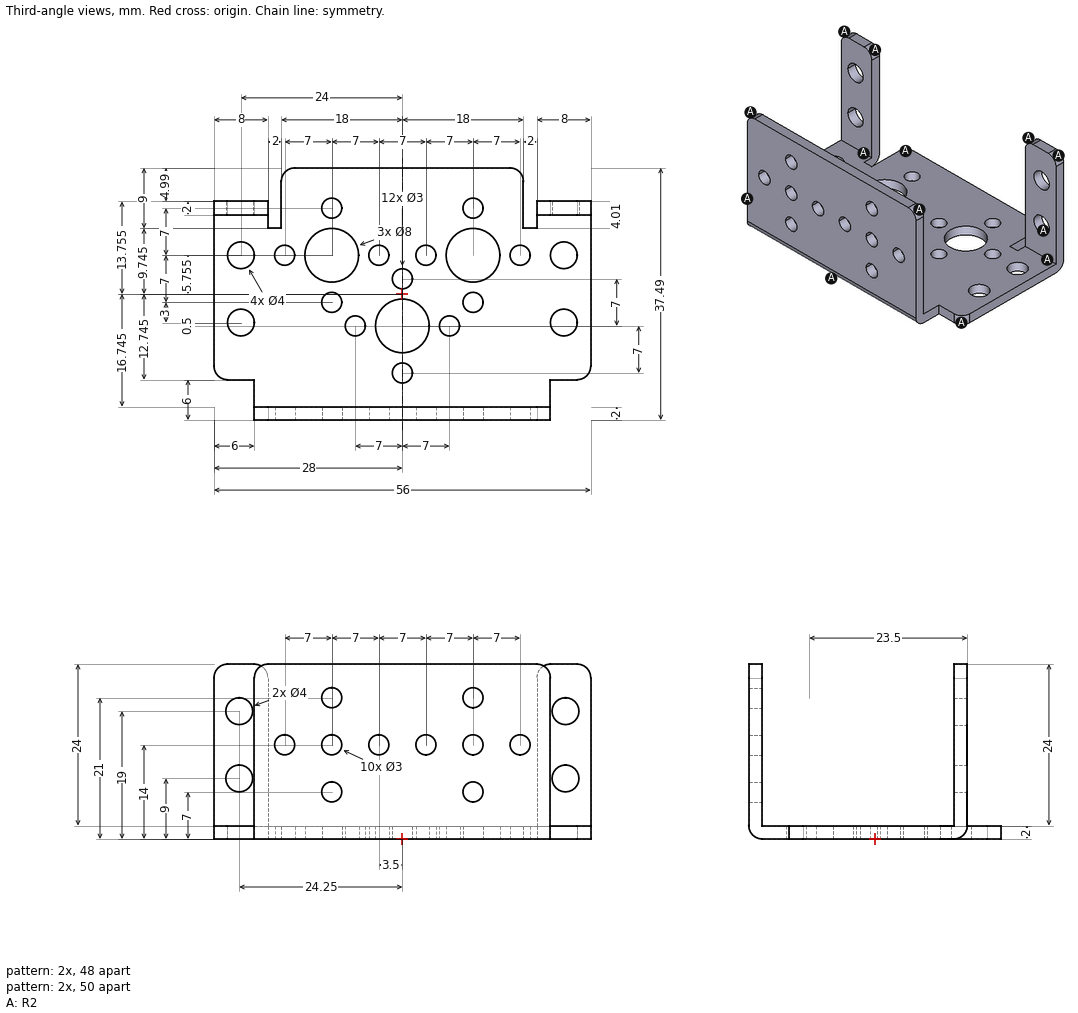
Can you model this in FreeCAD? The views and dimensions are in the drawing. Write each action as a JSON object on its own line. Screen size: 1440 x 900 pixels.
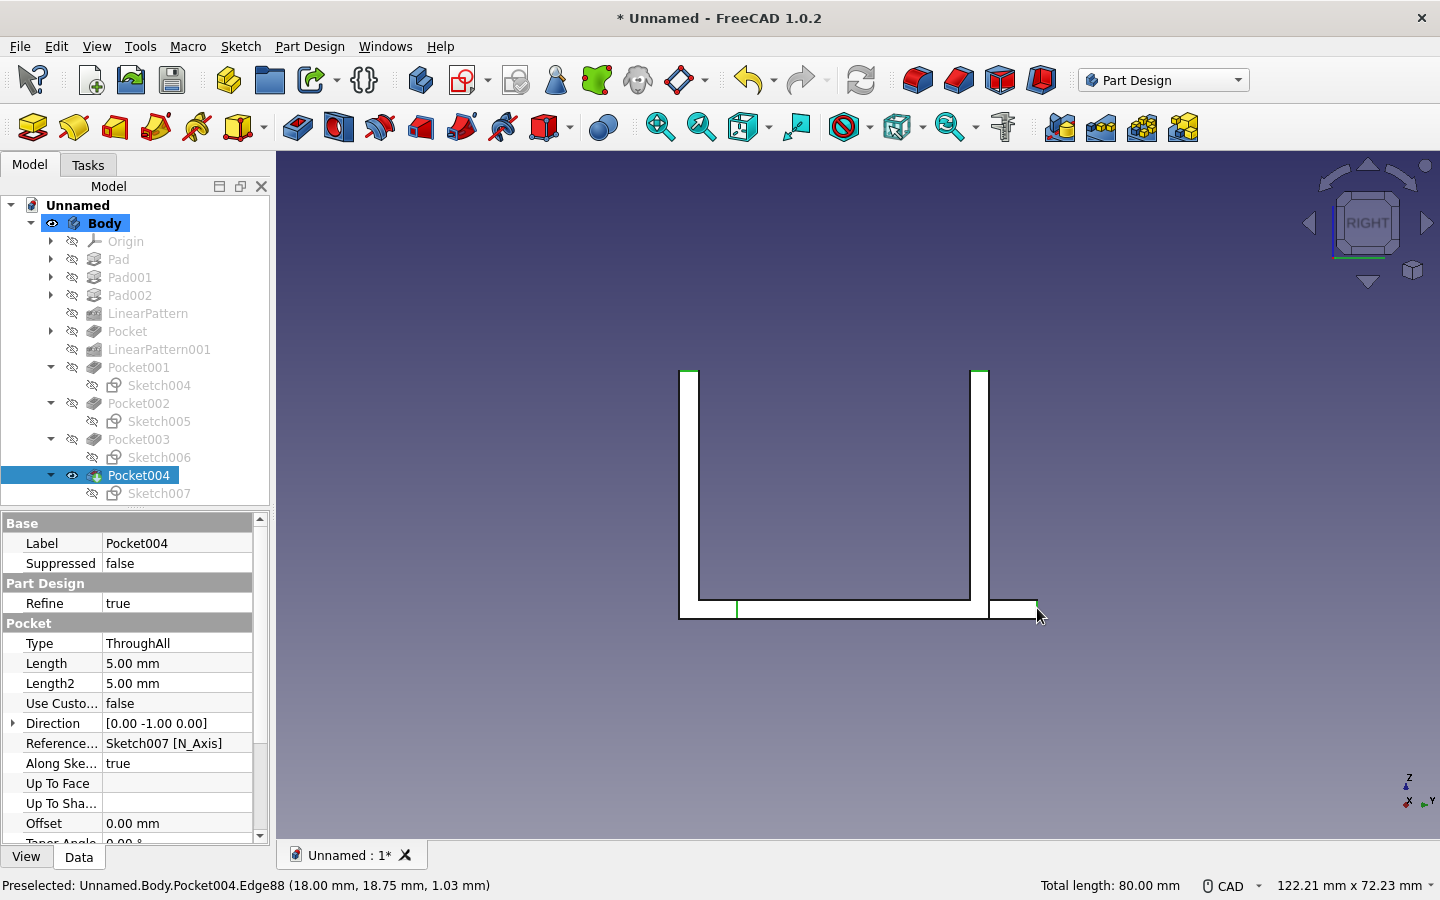
{"action": "left_click", "coordinate": [918, 80]}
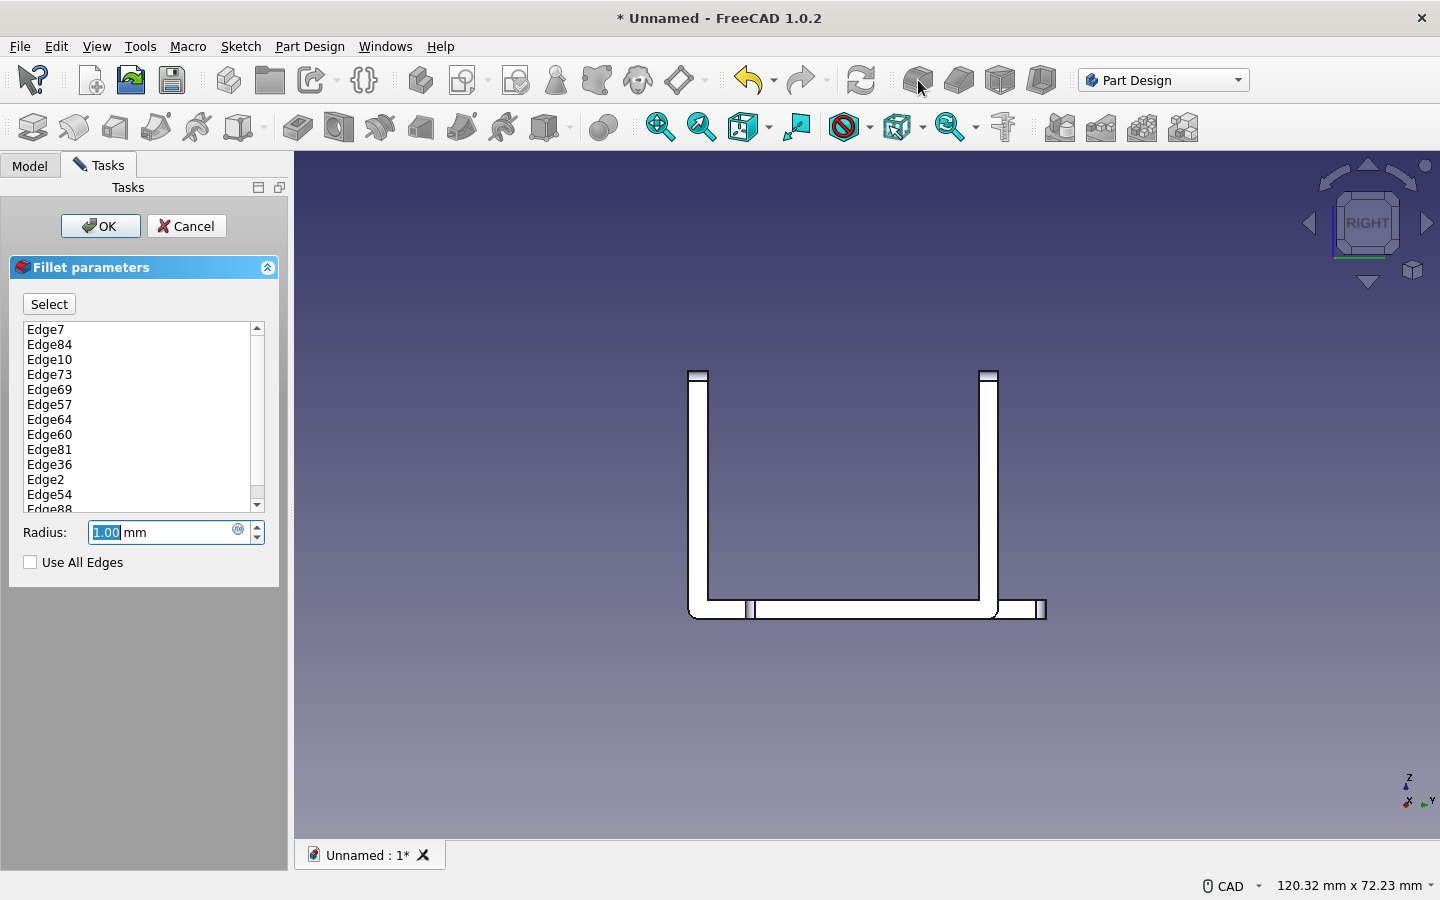
{"action": "type", "text": "2"}
{"action": "key", "text": "Tab"}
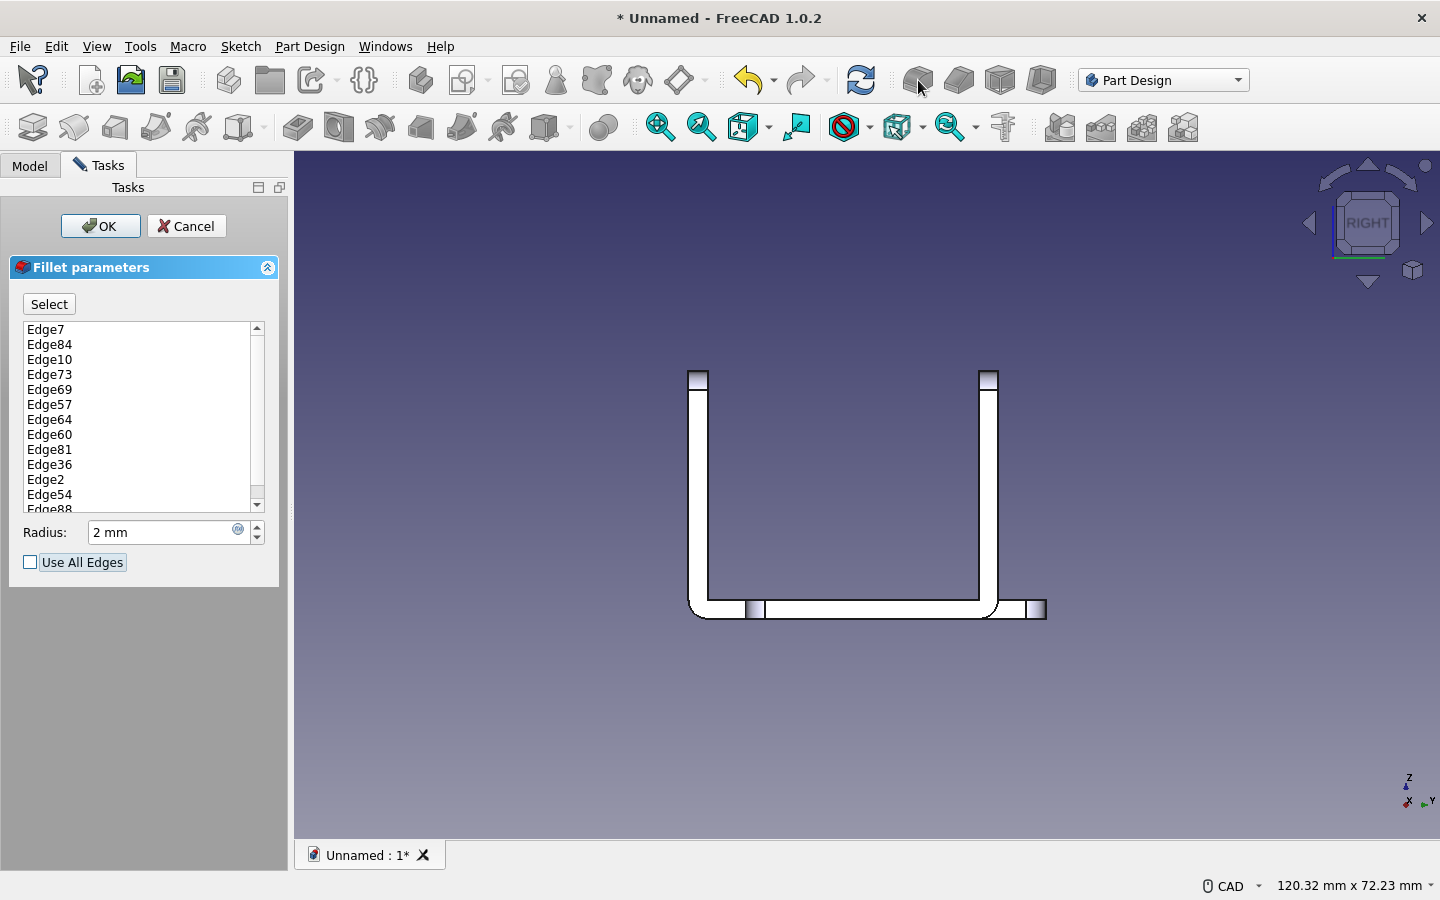
{"action": "left_click", "coordinate": [101, 226]}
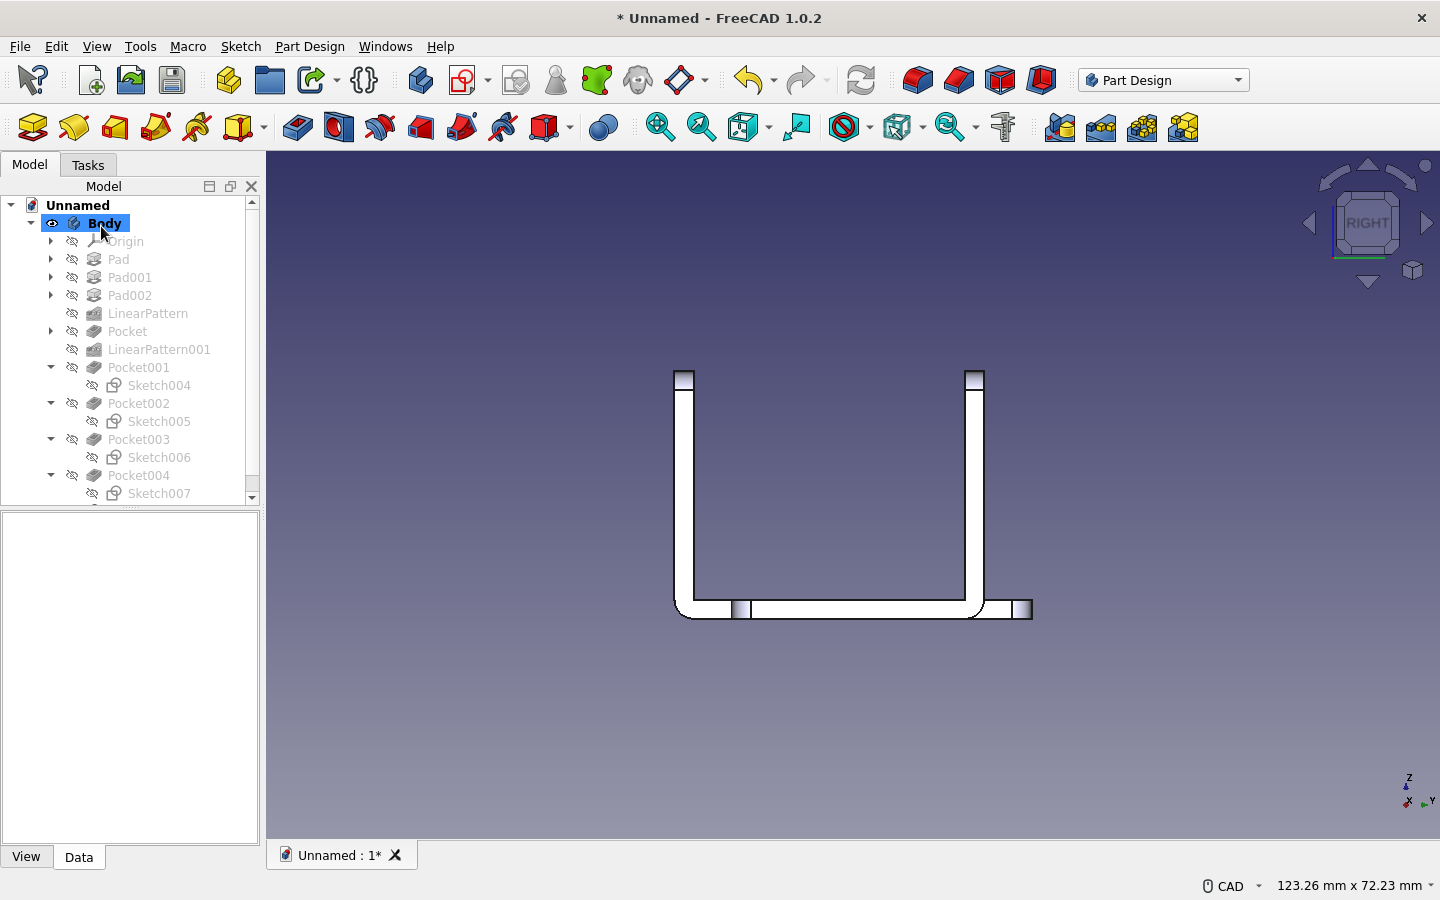
{"action": "key", "text": "v f"}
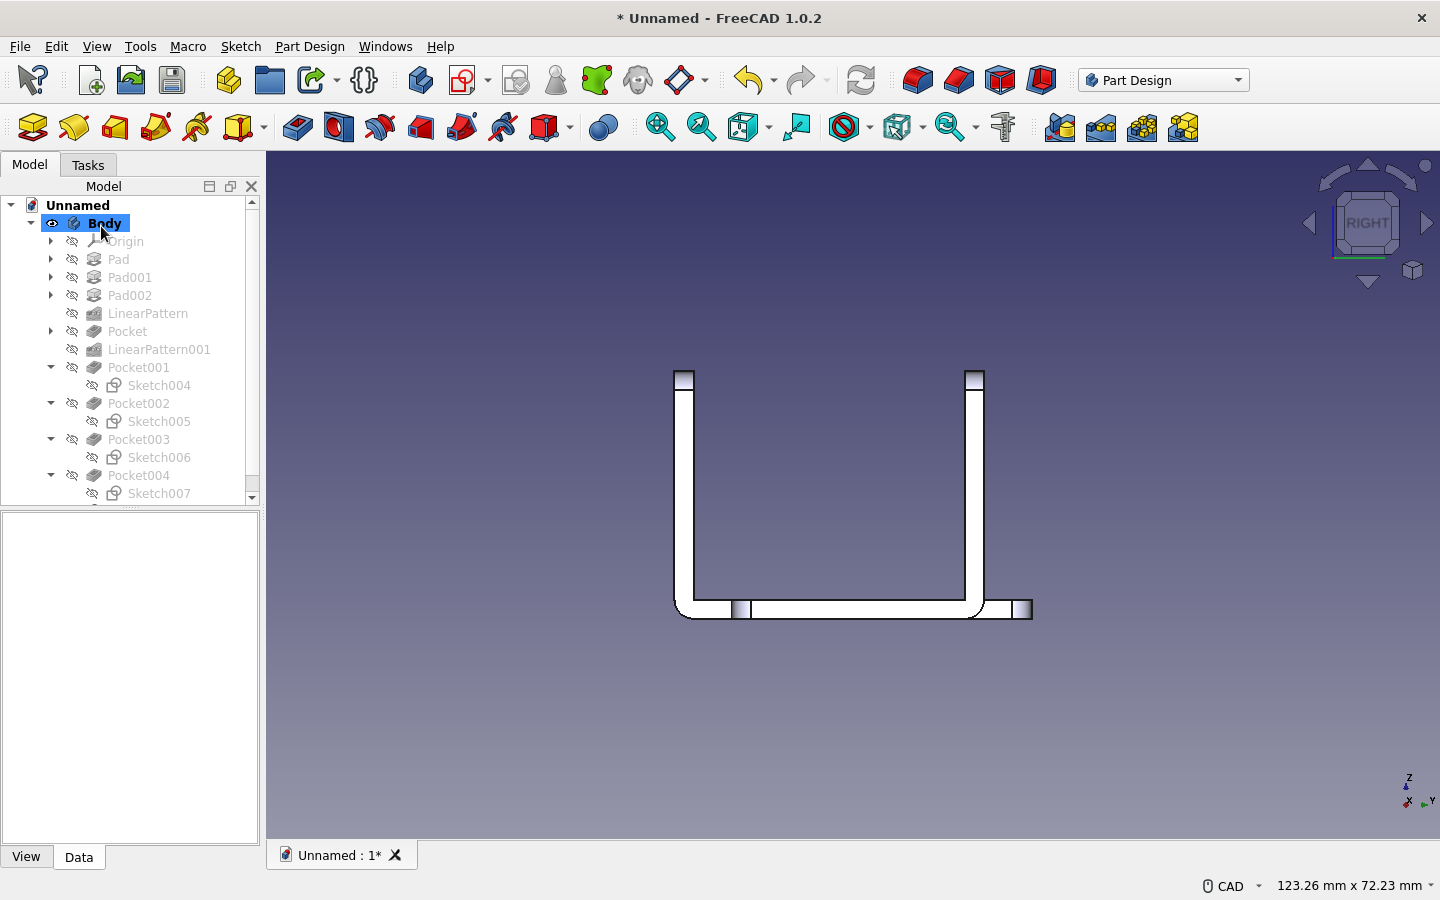
{"action": "key", "text": "4"}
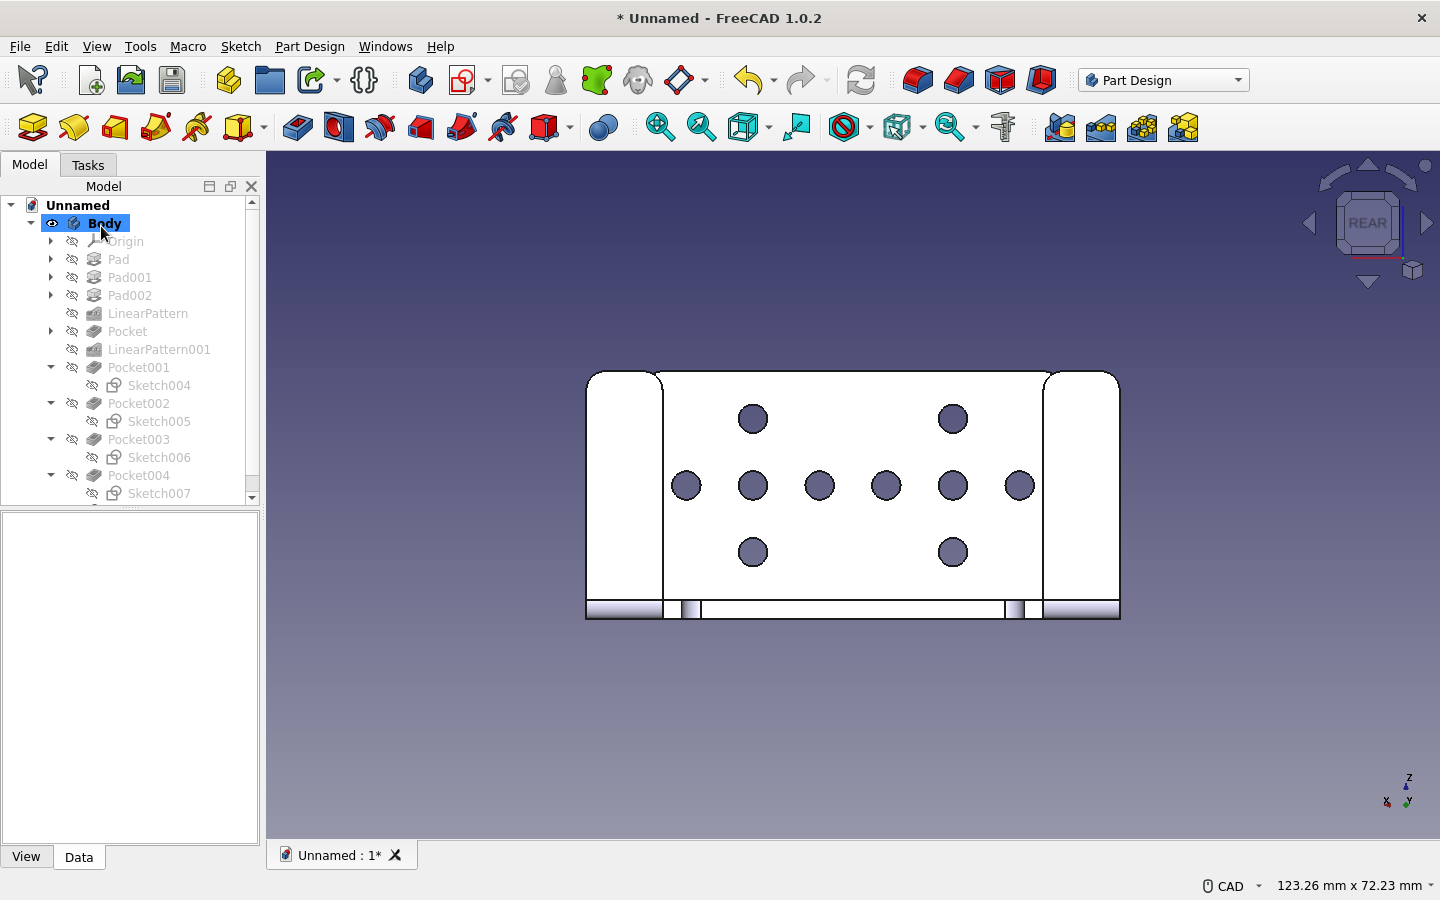
{"action": "left_click", "coordinate": [624, 419]}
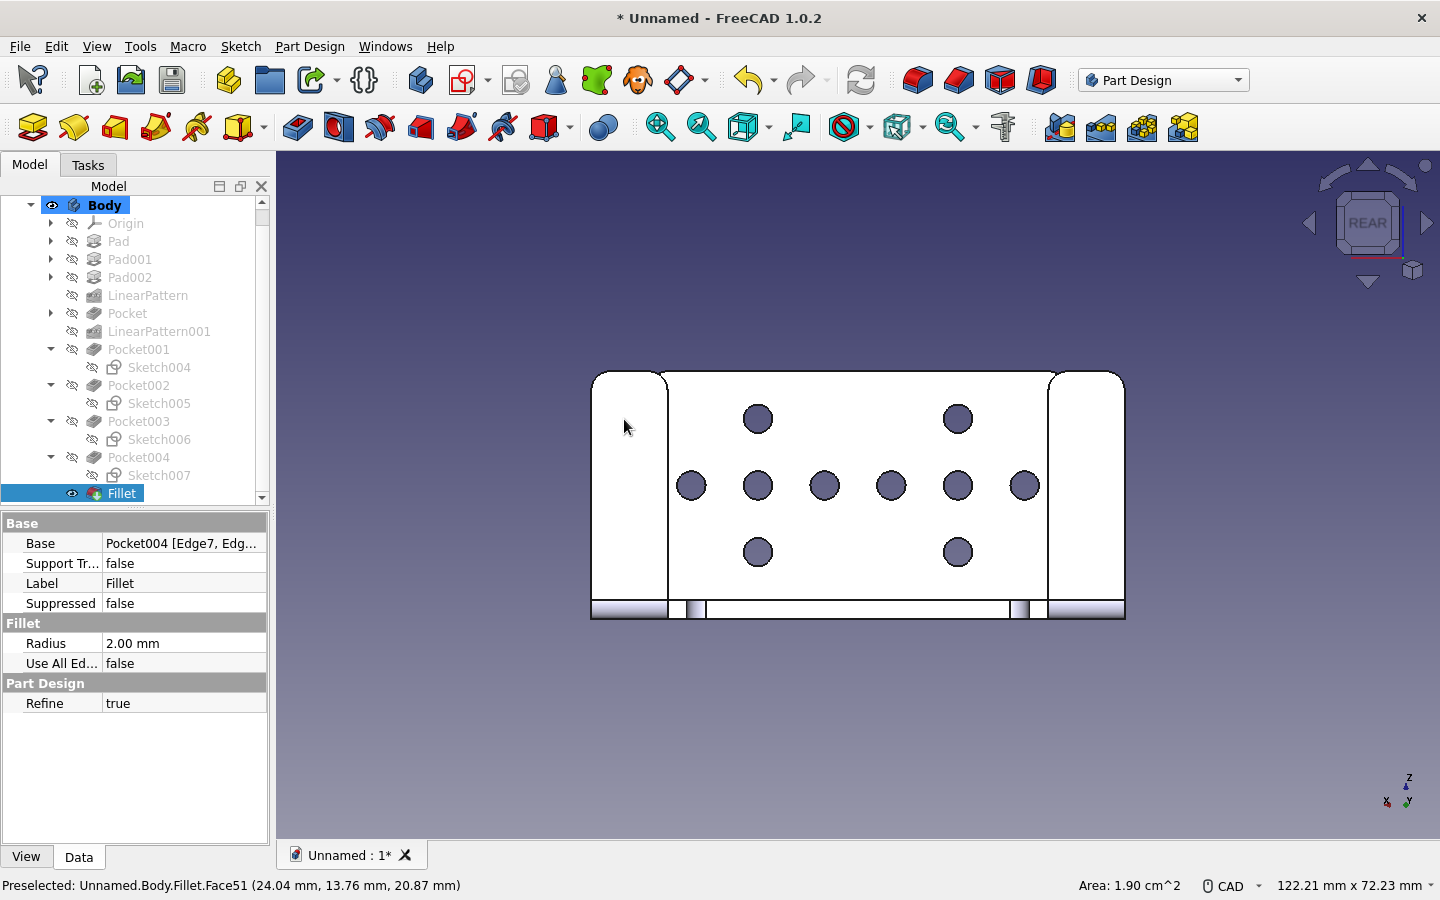
{"action": "left_click", "coordinate": [462, 80]}